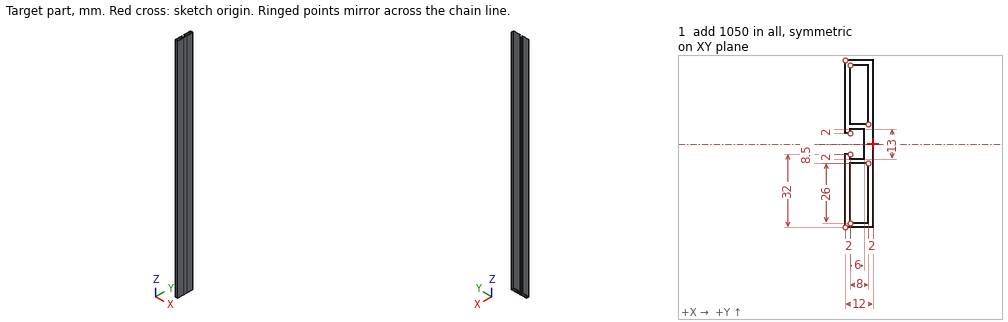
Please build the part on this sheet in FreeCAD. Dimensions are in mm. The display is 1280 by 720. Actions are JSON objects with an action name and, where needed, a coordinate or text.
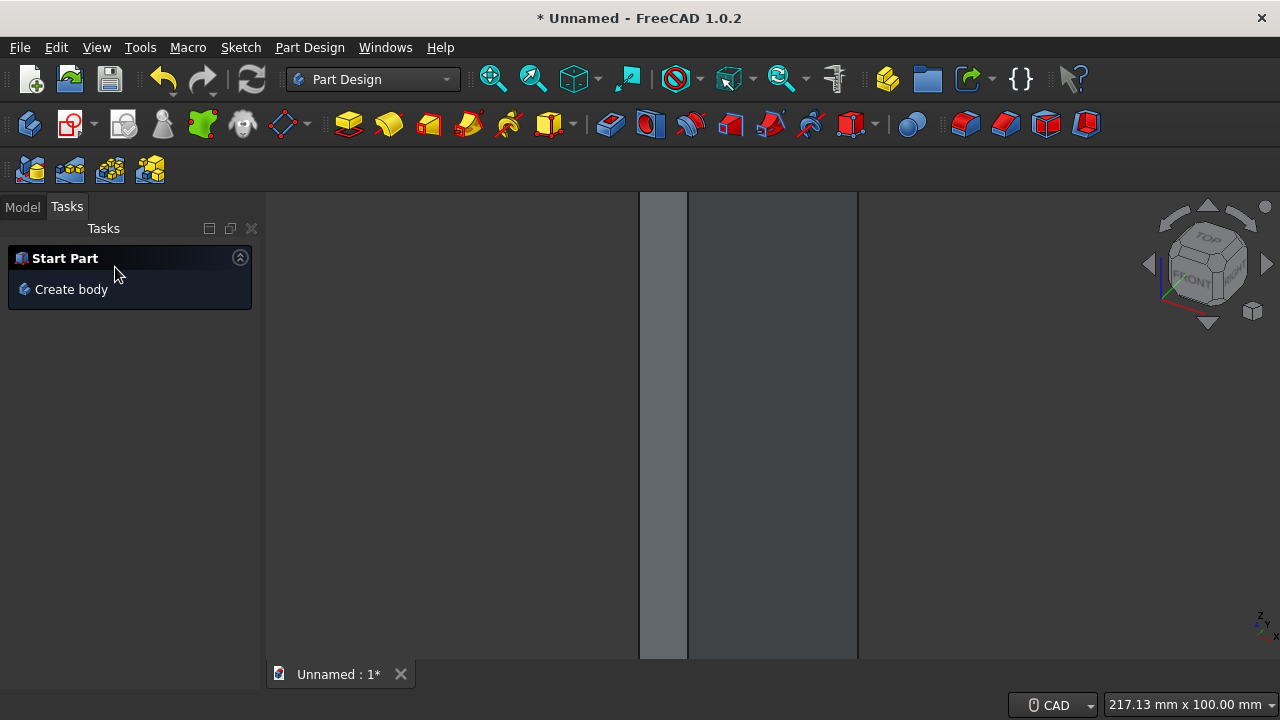
{"action": "key", "text": "0"}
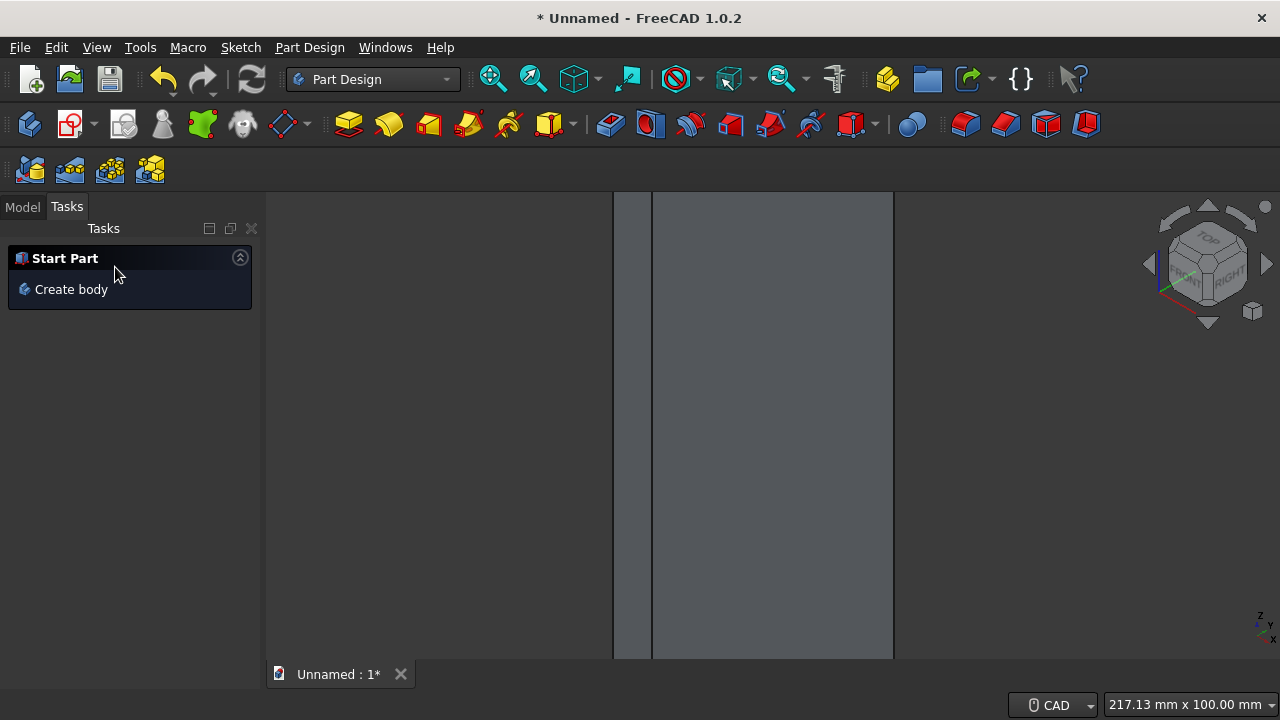
{"action": "left_click", "coordinate": [494, 80]}